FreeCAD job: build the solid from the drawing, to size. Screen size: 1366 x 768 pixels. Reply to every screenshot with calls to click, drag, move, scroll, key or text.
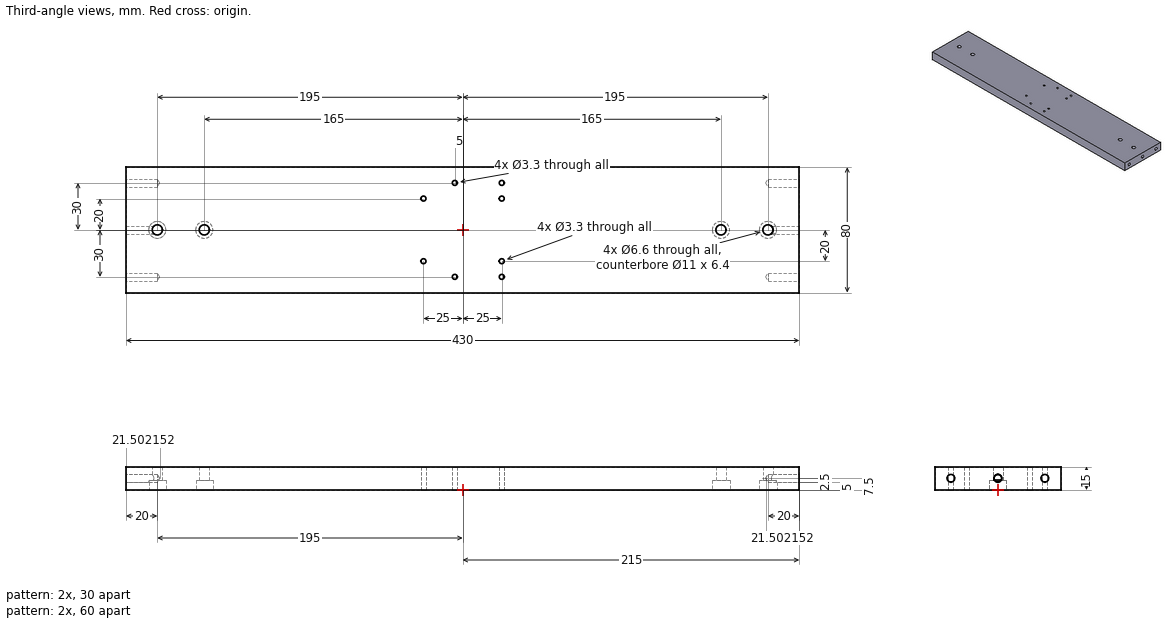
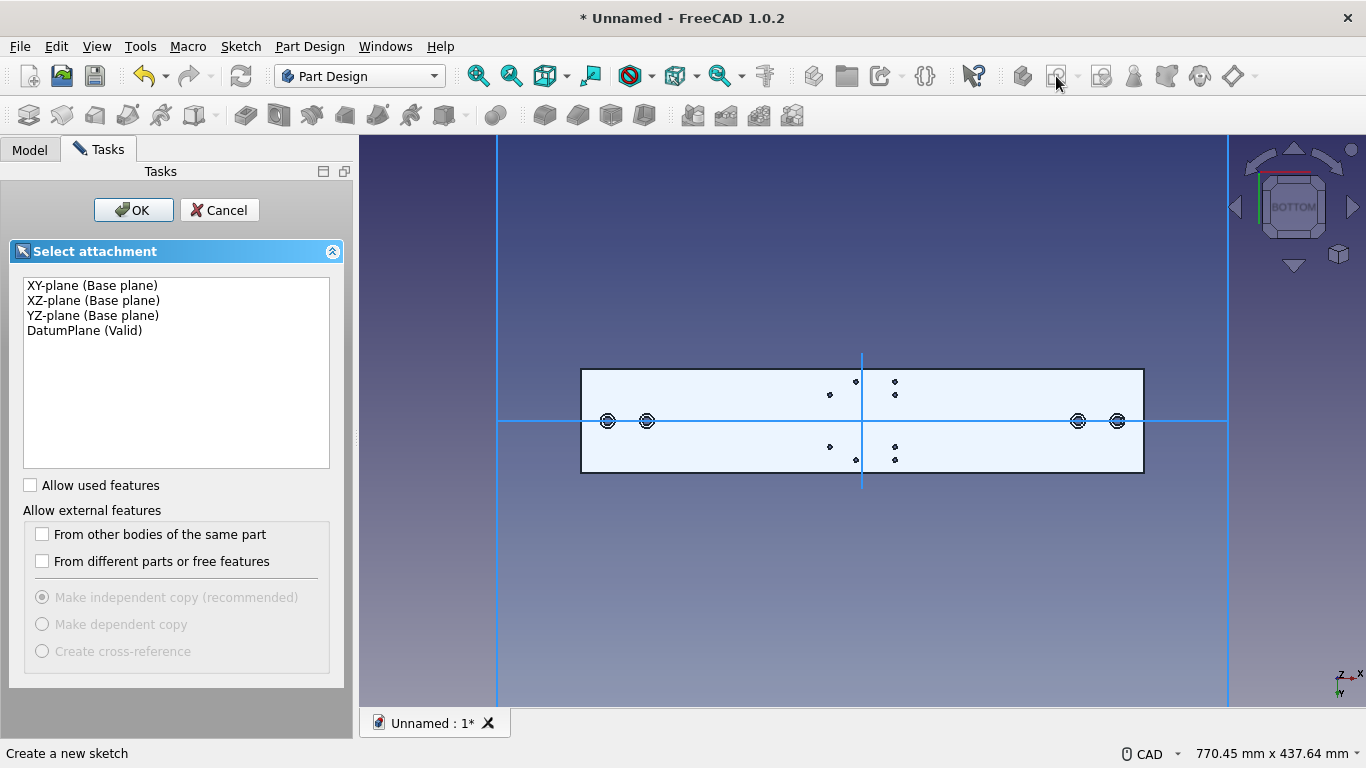
click(84, 300)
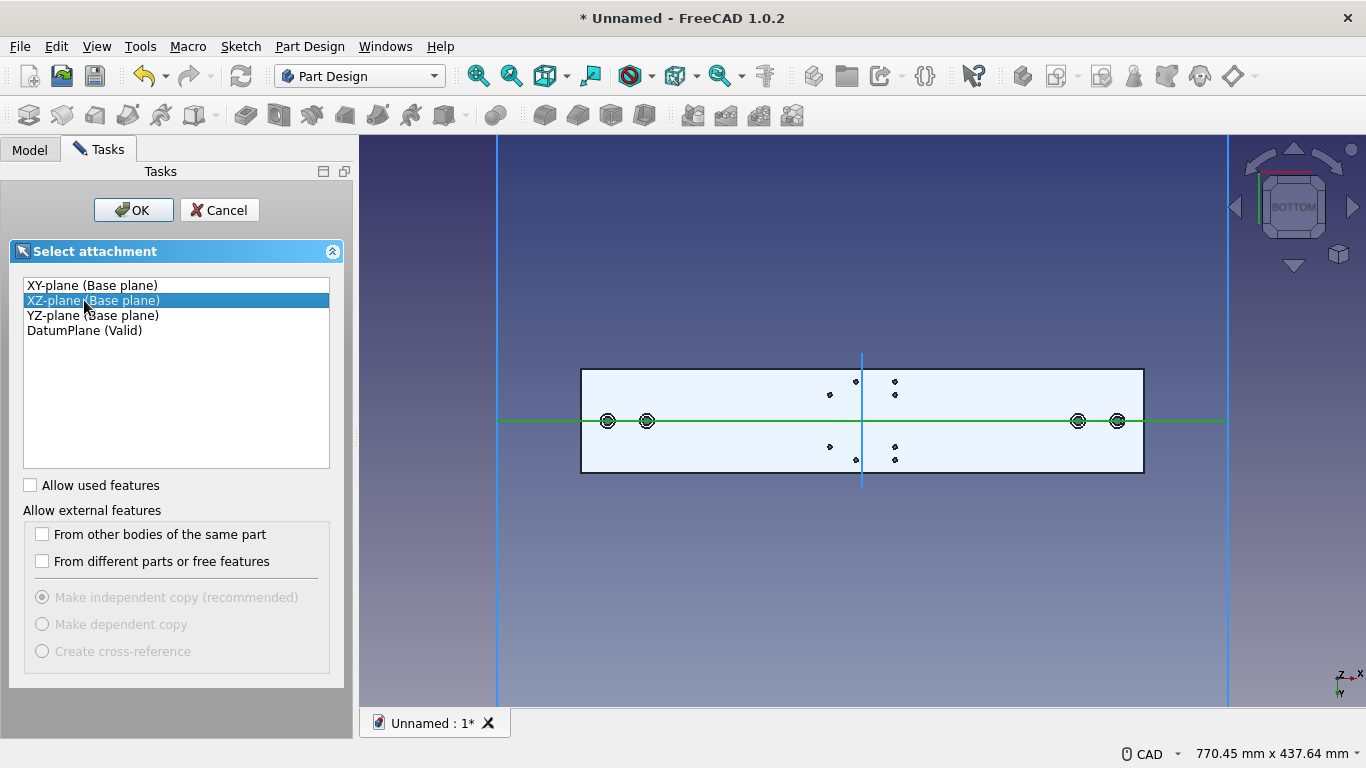
click(134, 210)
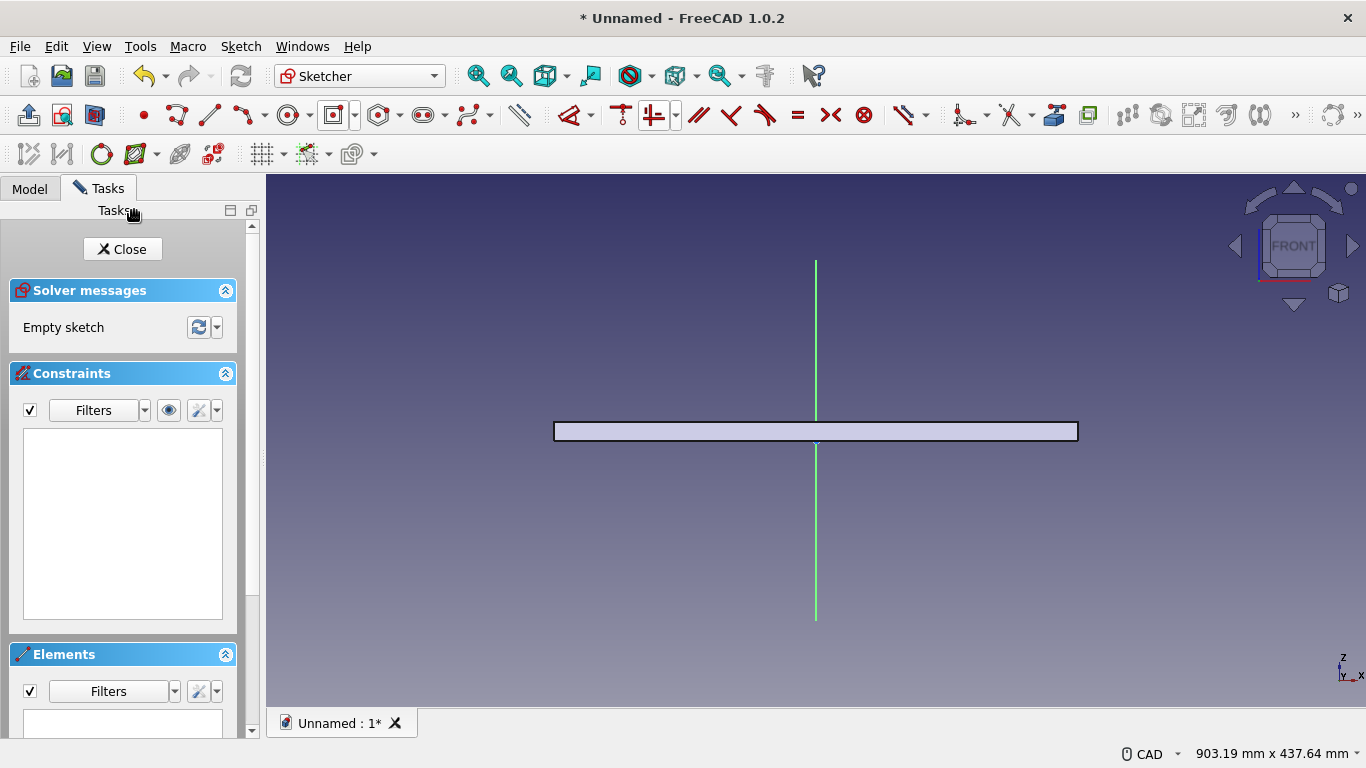
click(95, 116)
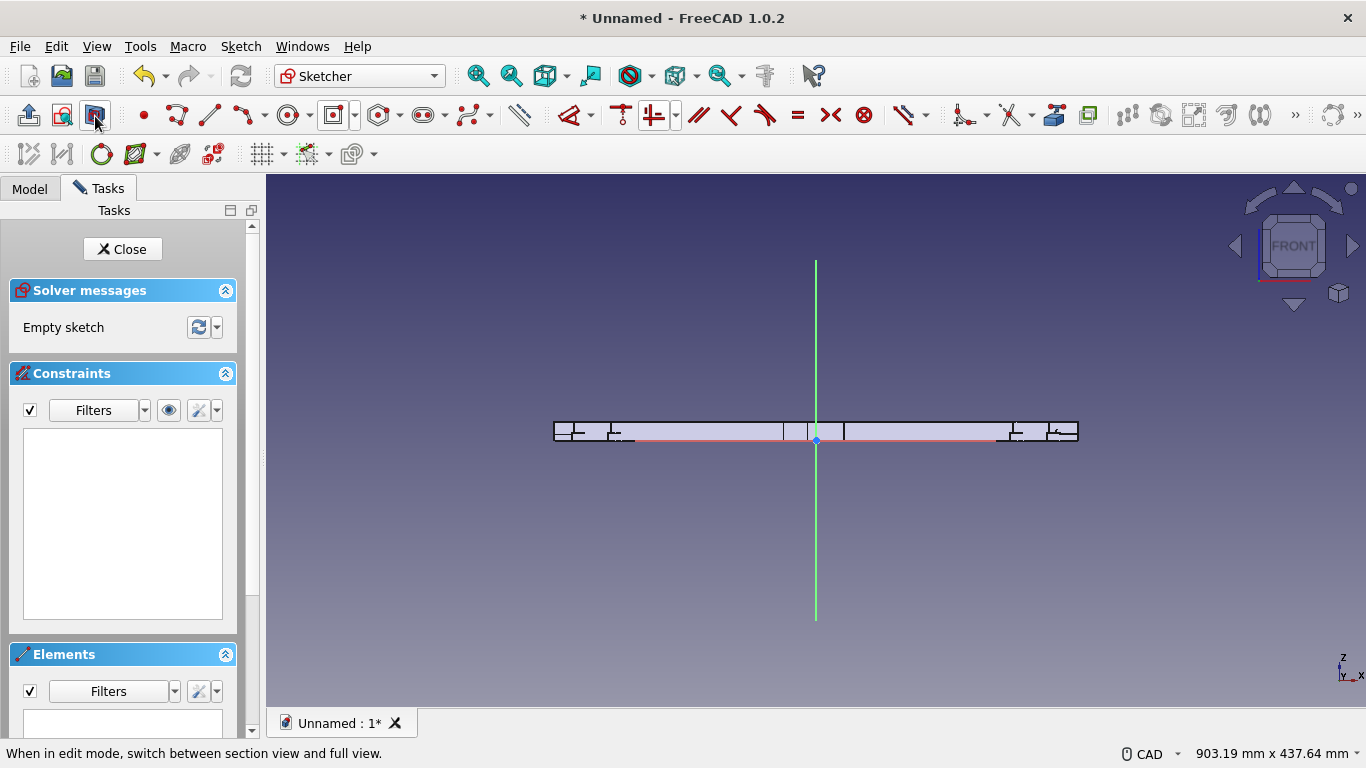
scroll(550, 432, up, 14)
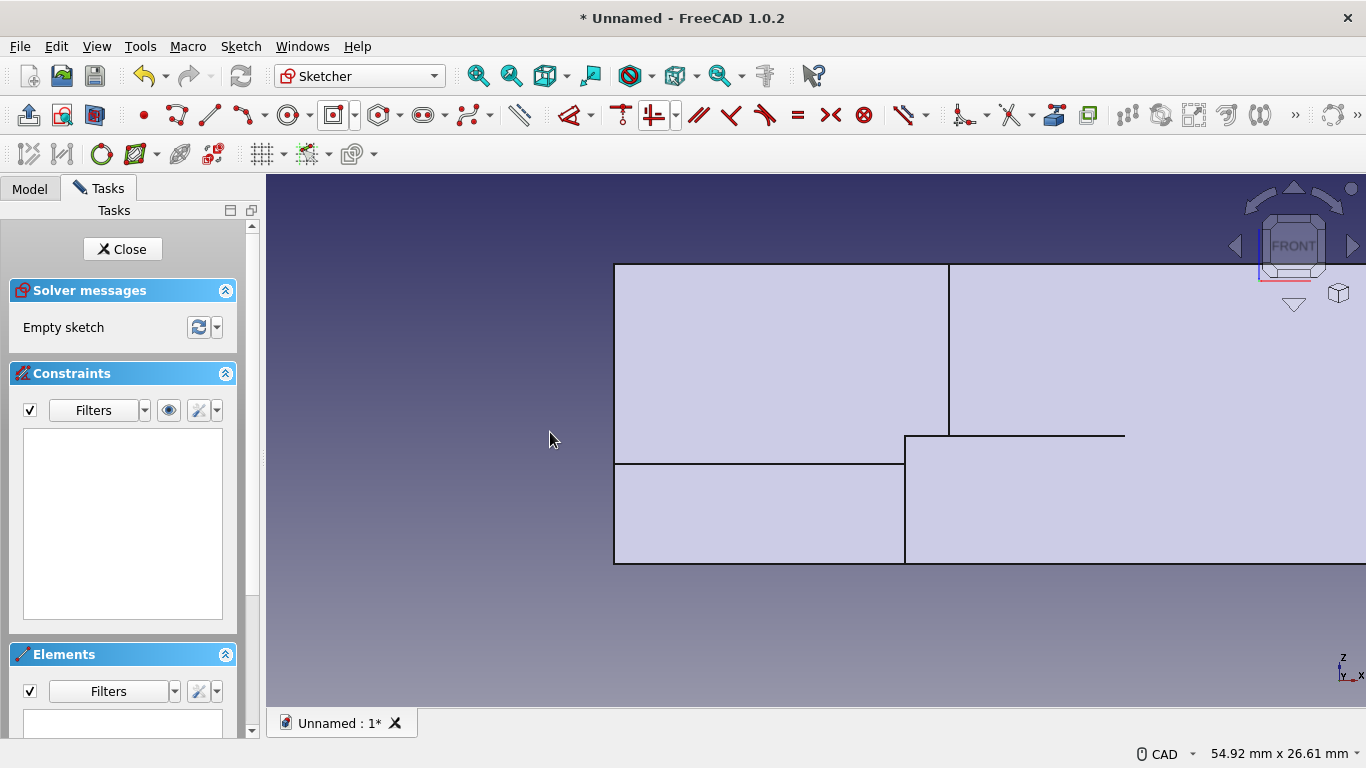
click(177, 116)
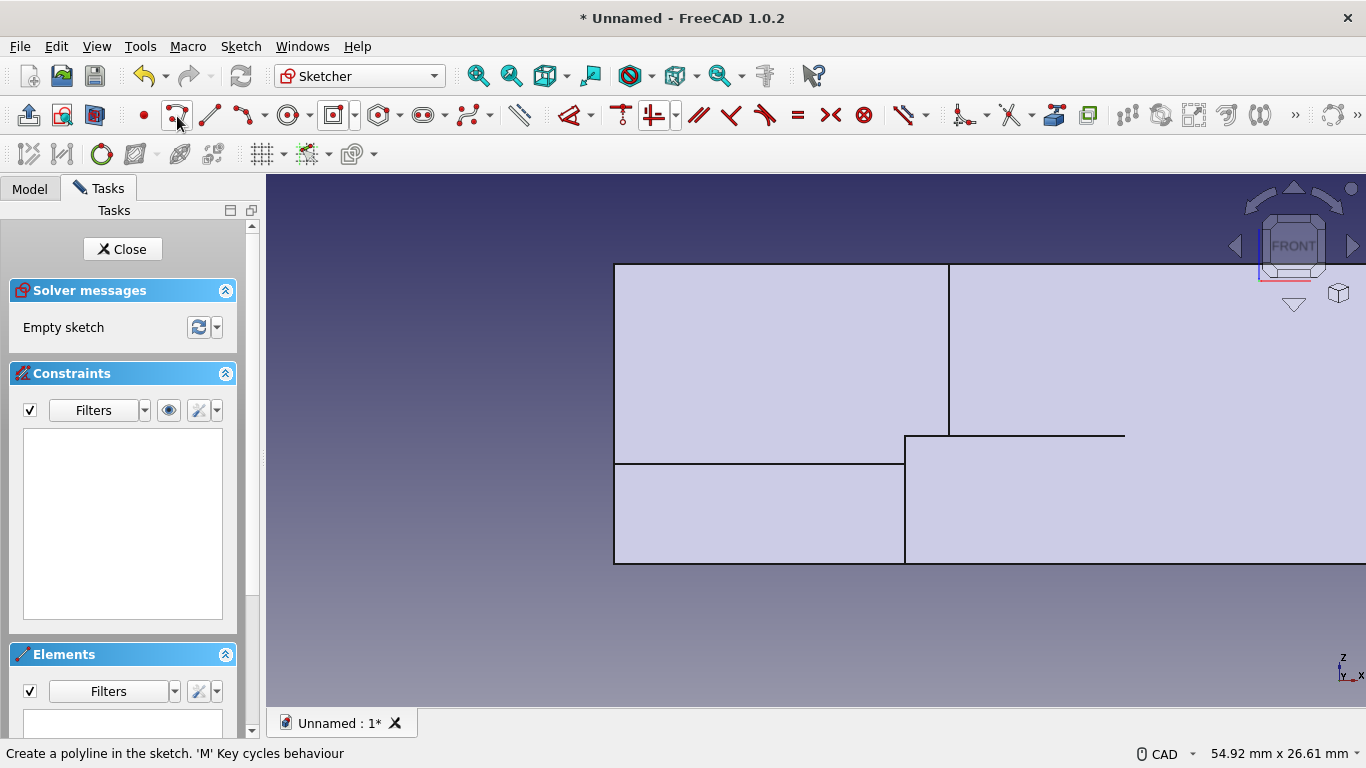
click(1045, 414)
click(1015, 464)
click(614, 464)
click(614, 414)
click(1045, 415)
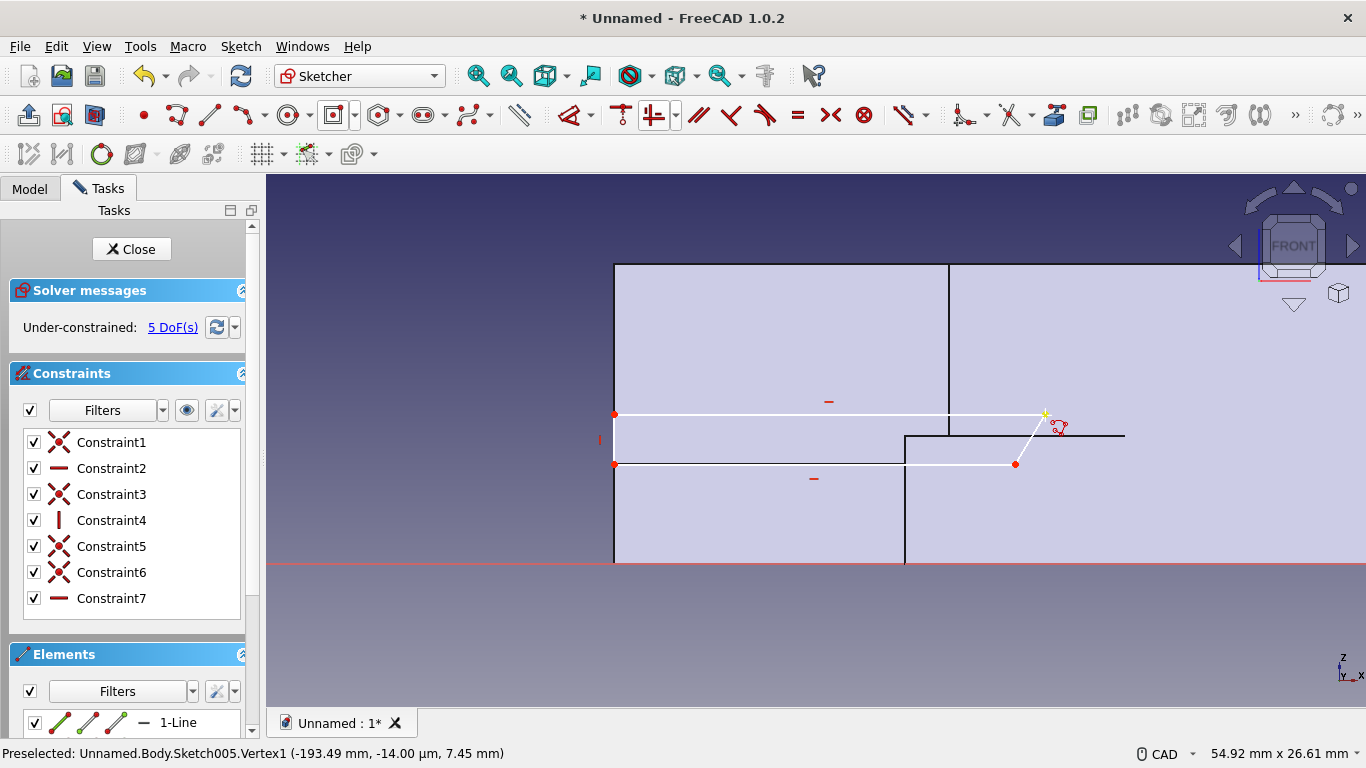
click(210, 116)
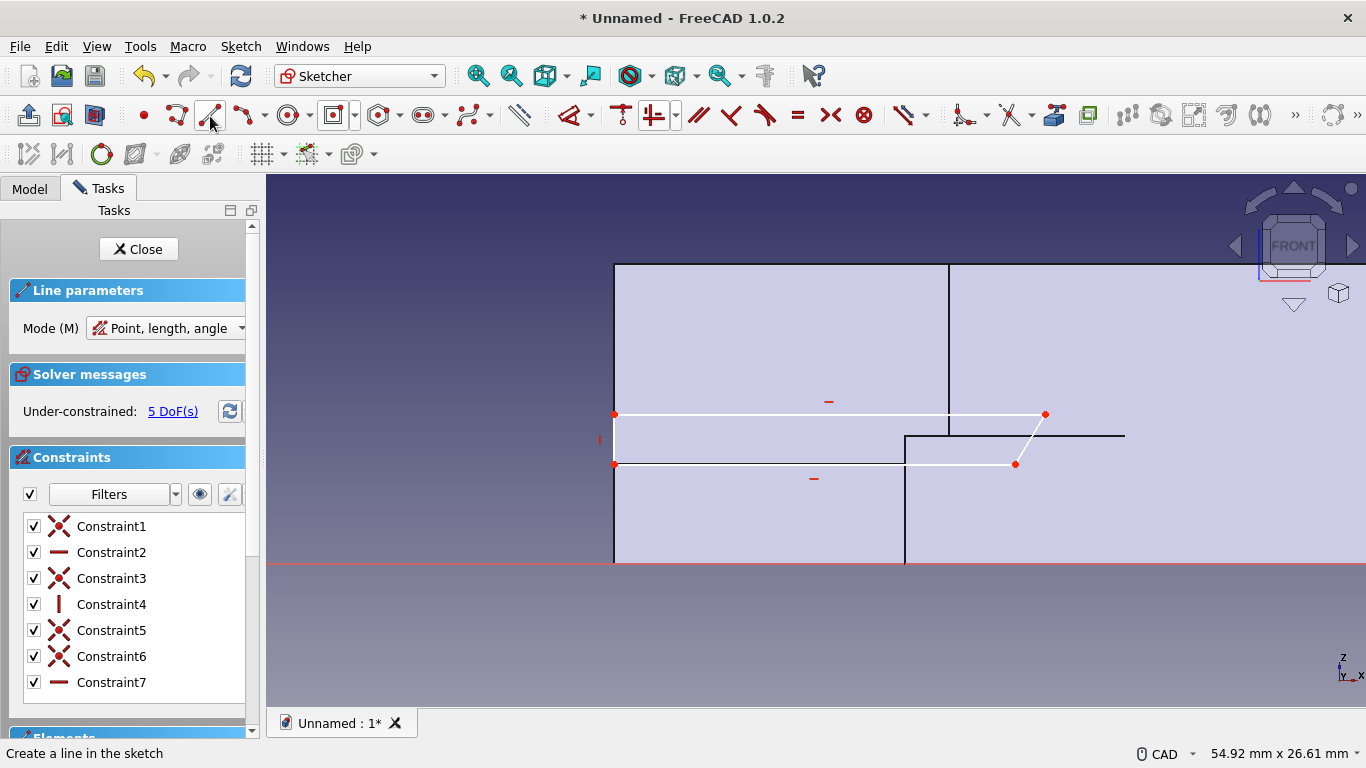
click(571, 414)
click(442, 414)
key(Escape)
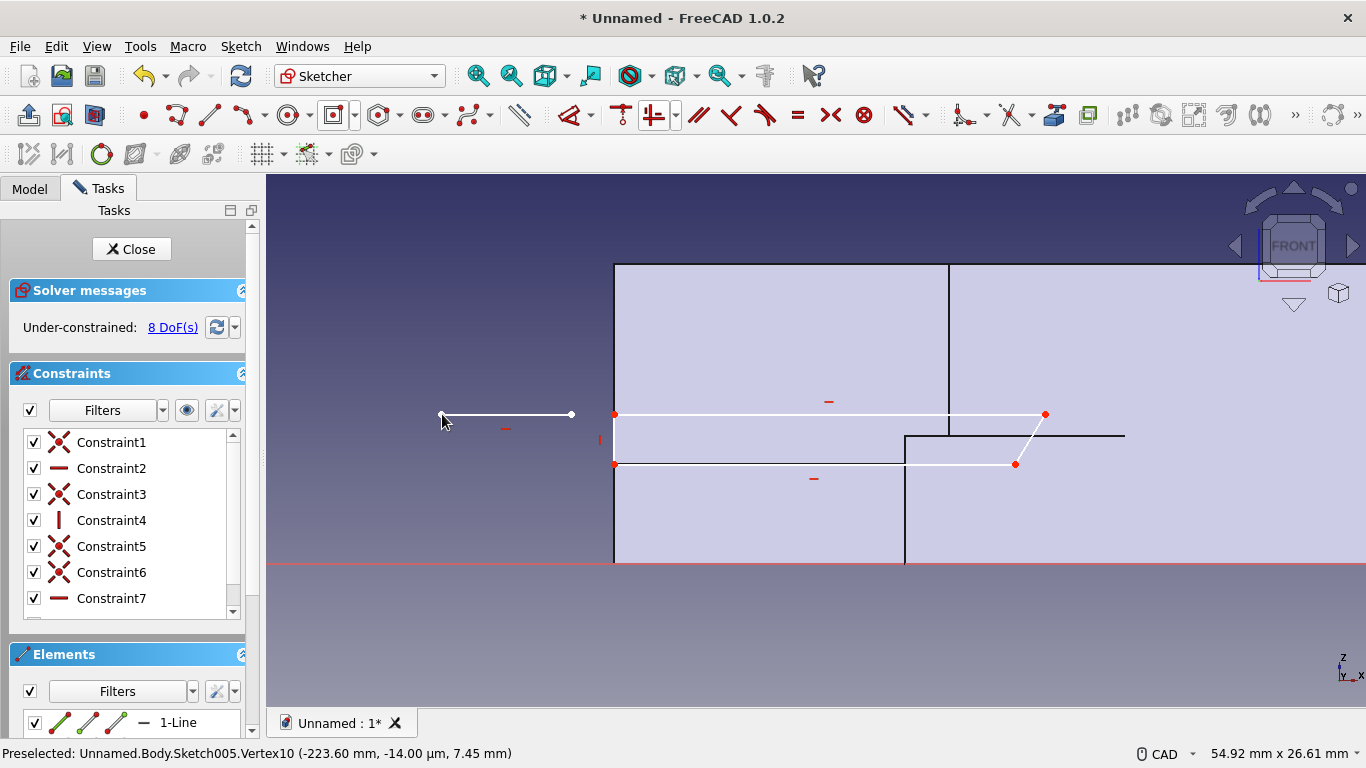
click(532, 415)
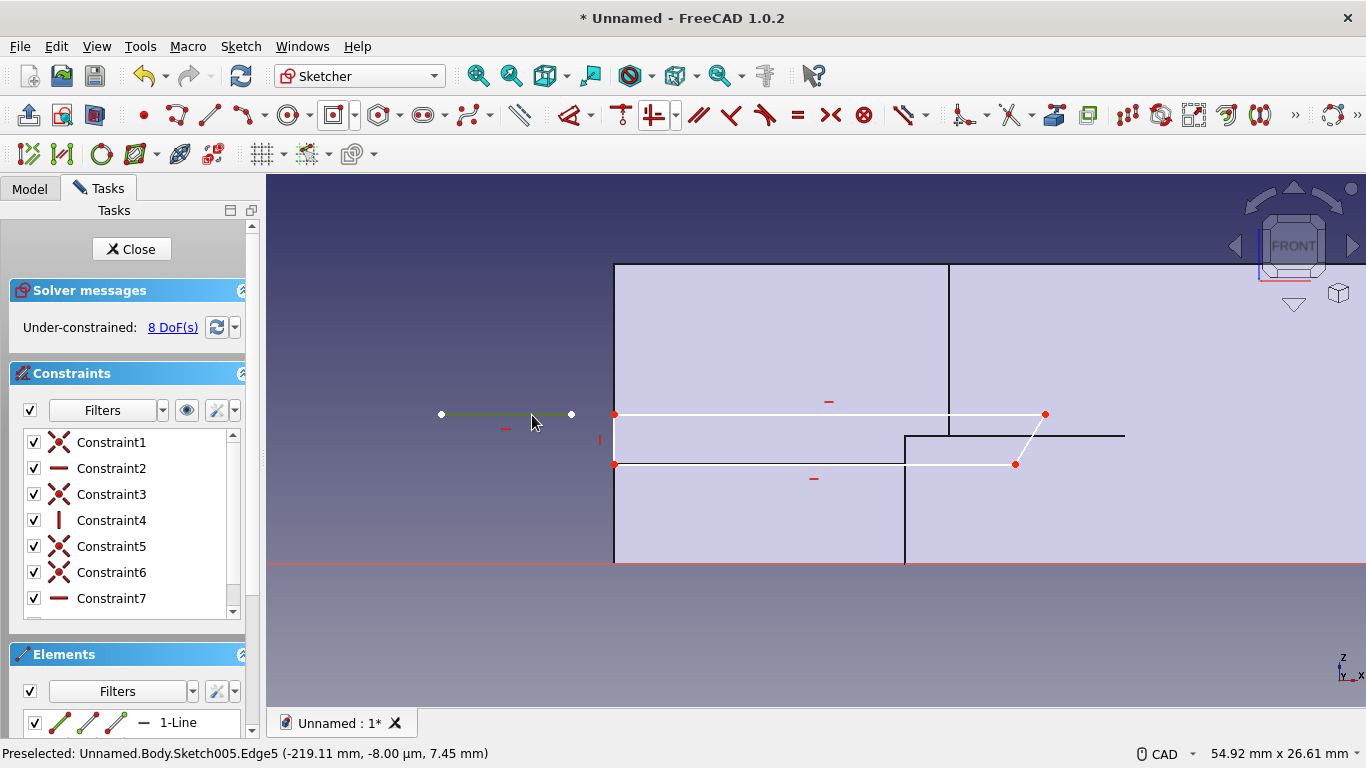
click(520, 116)